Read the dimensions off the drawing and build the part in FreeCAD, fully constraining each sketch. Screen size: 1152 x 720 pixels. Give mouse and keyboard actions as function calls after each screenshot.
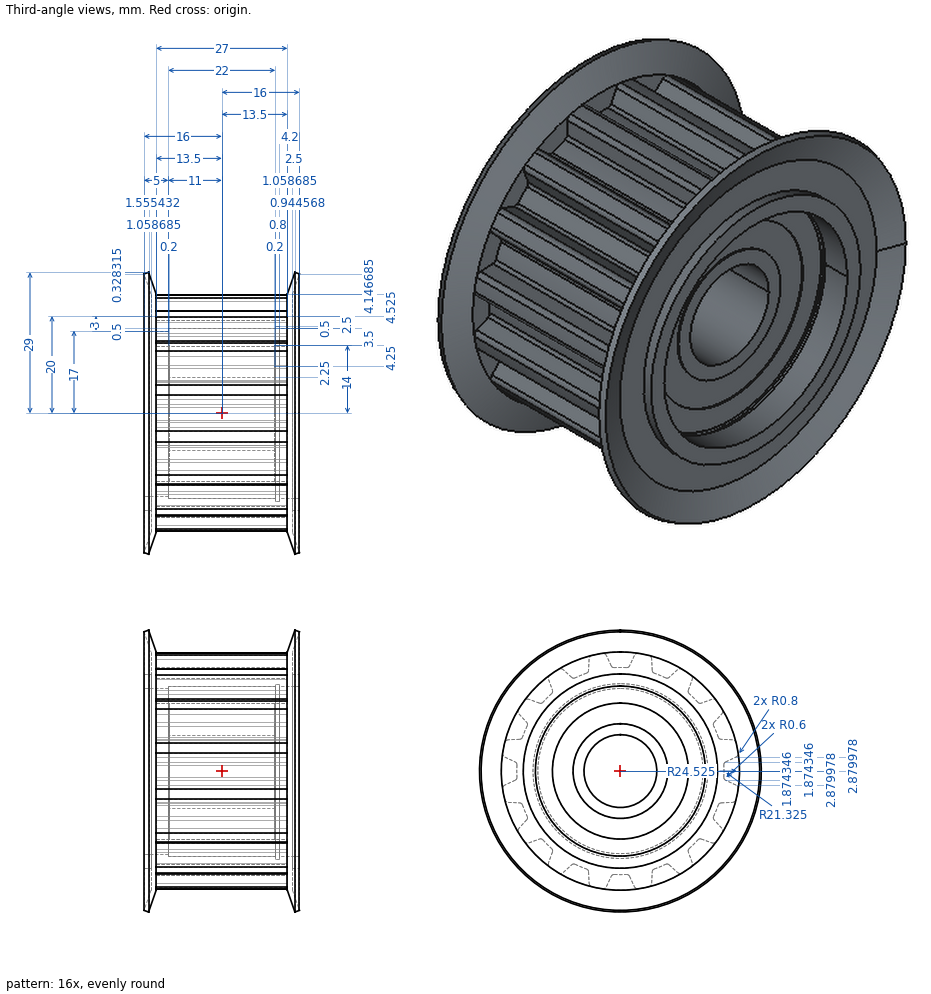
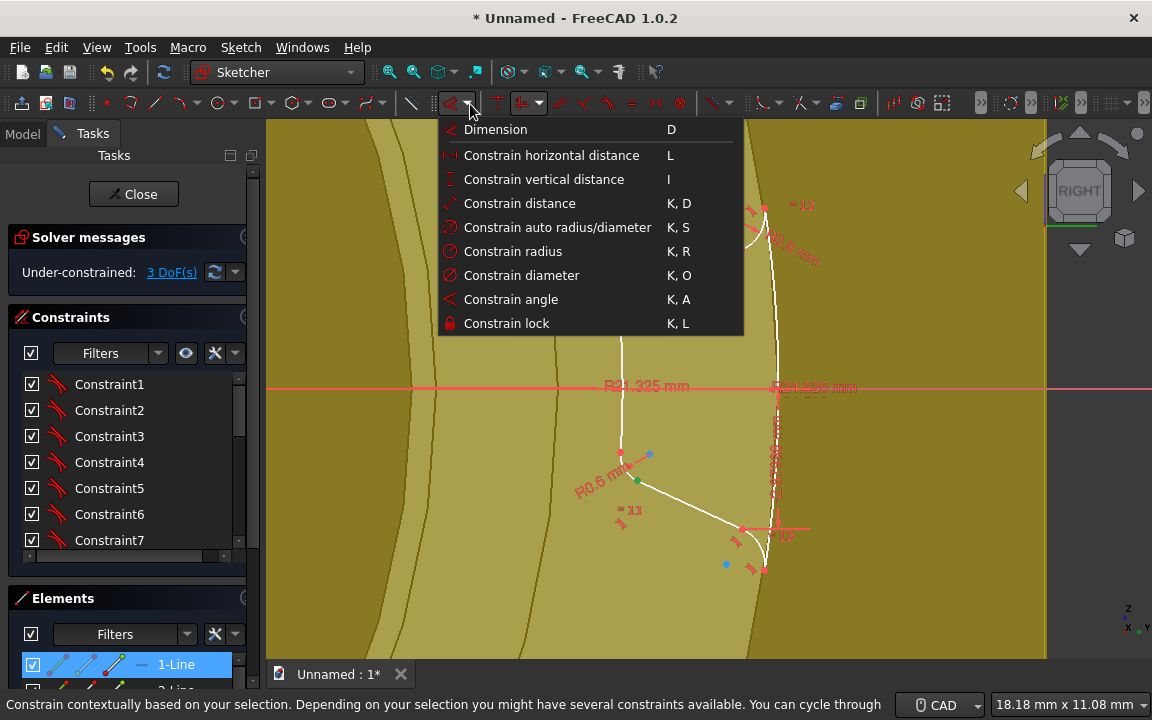
click(591, 179)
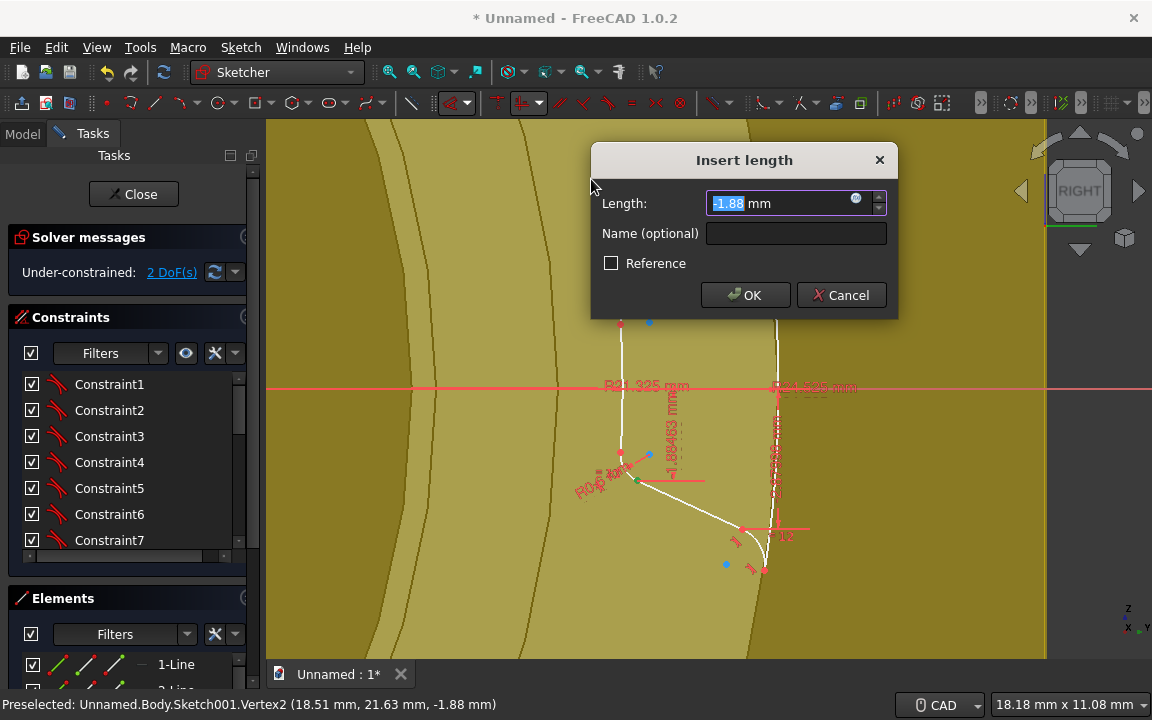
text(-1.874346)
key(Return)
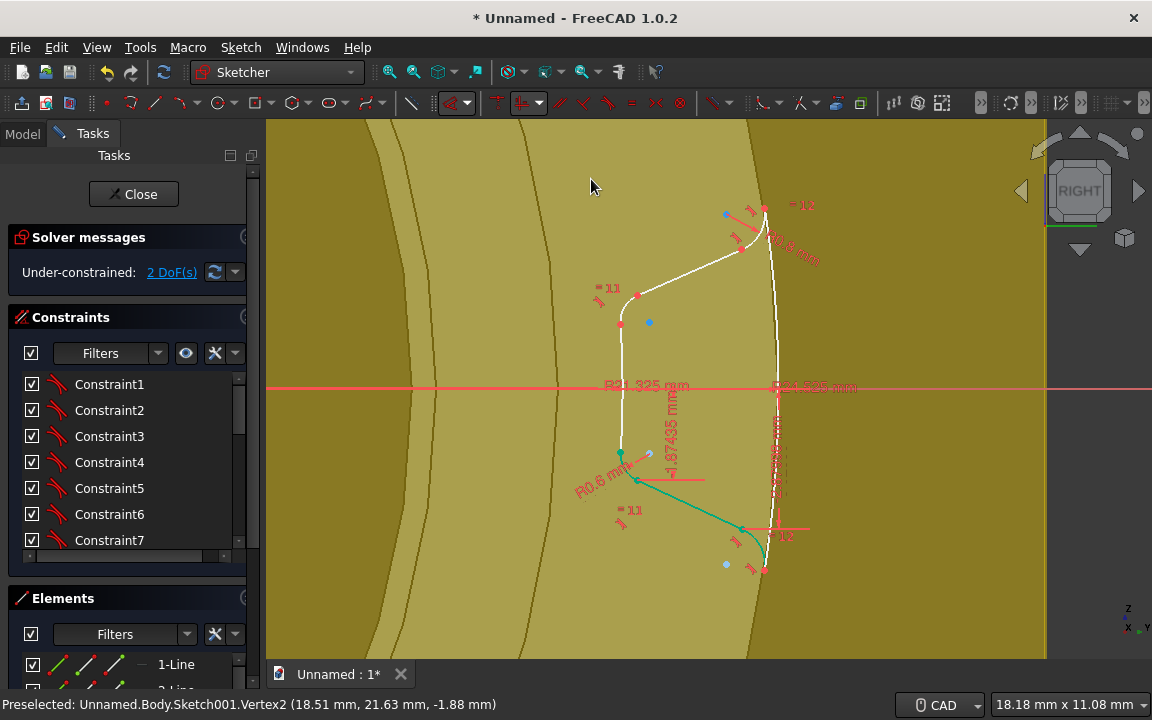
click(638, 295)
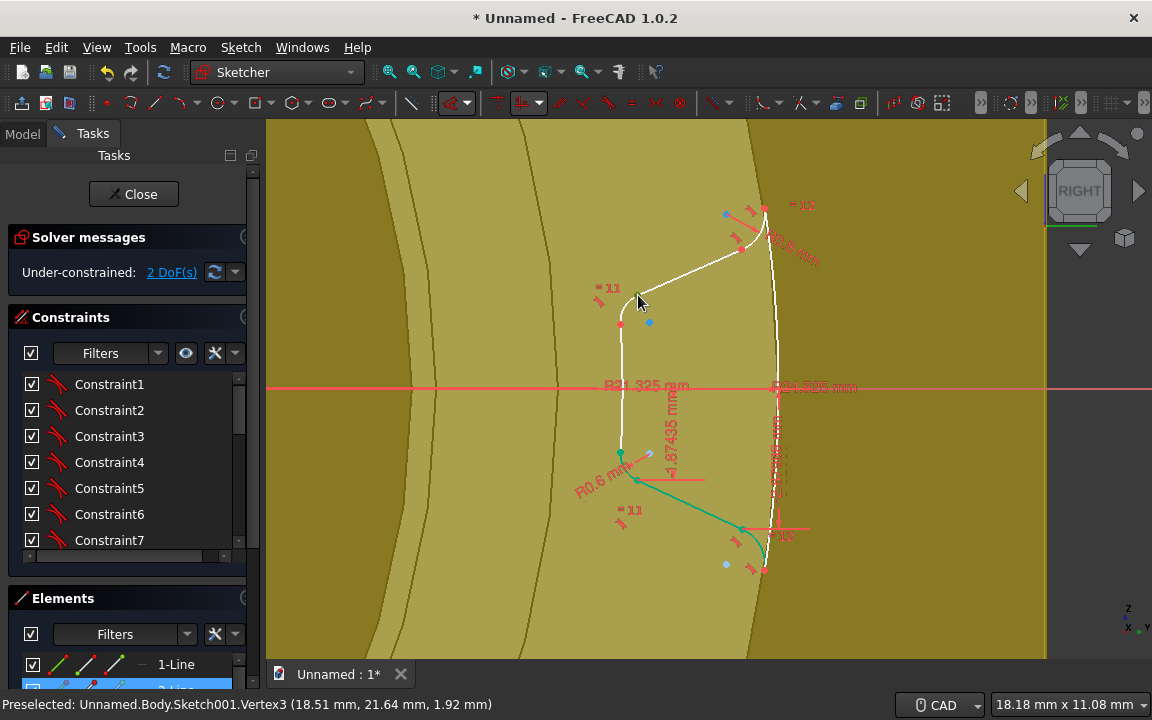
key(i)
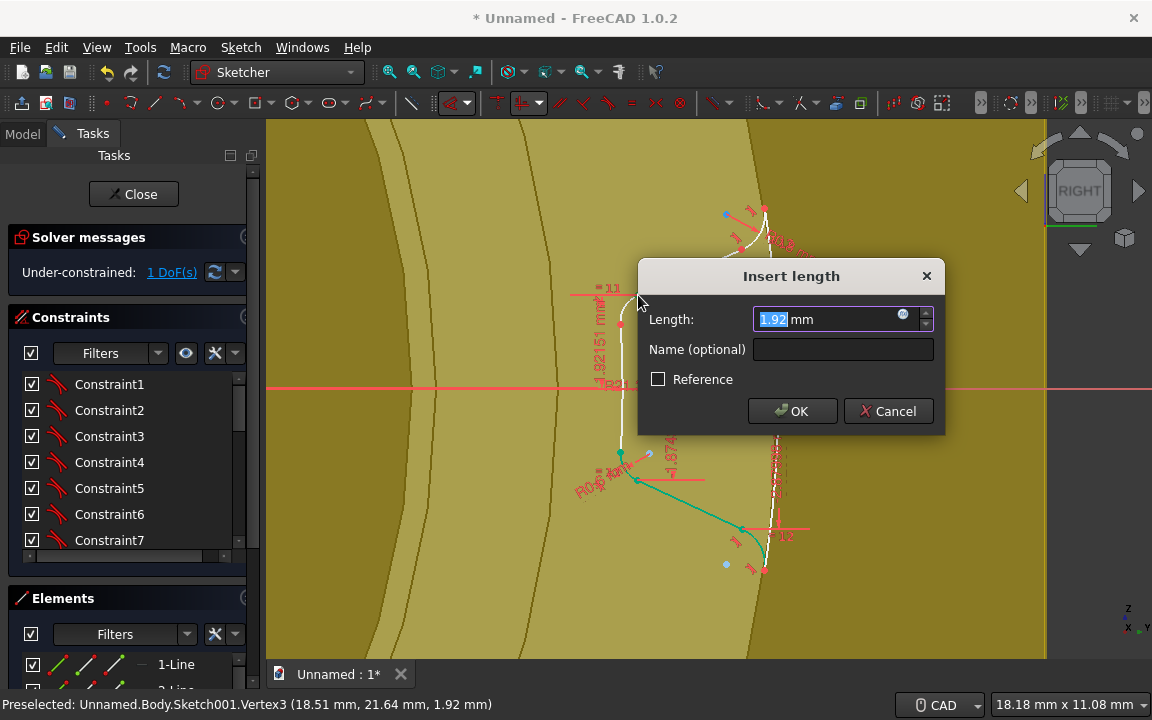
text(1.874346)
key(Return)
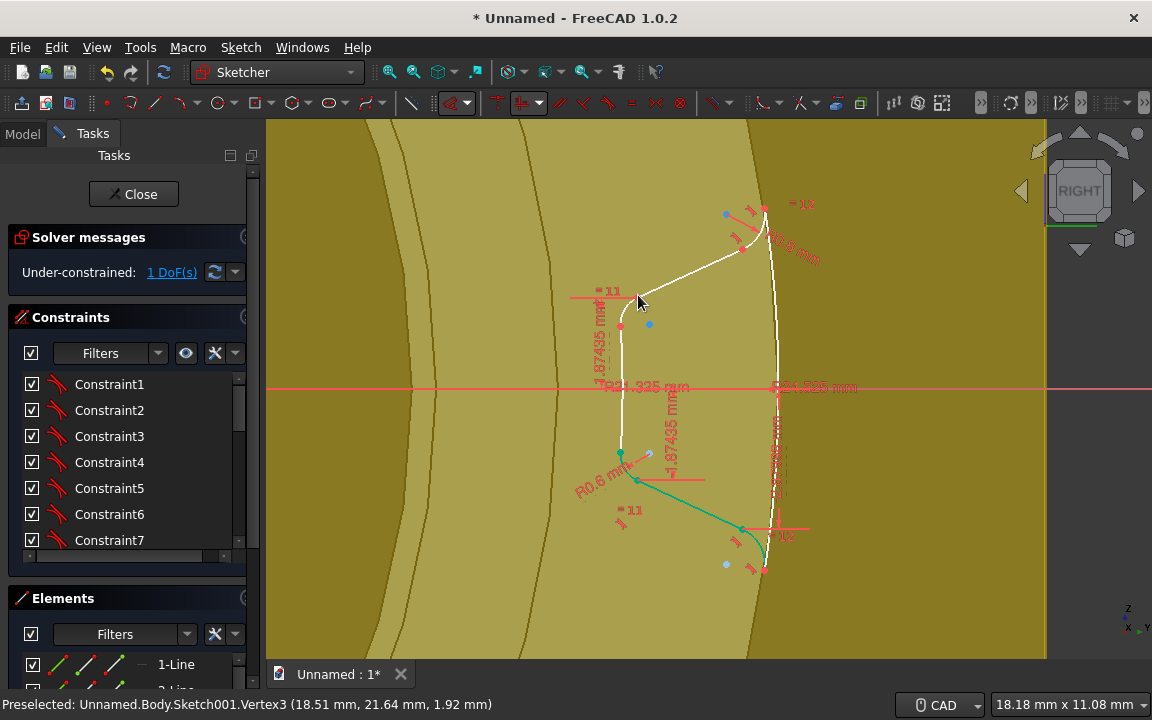
click(742, 250)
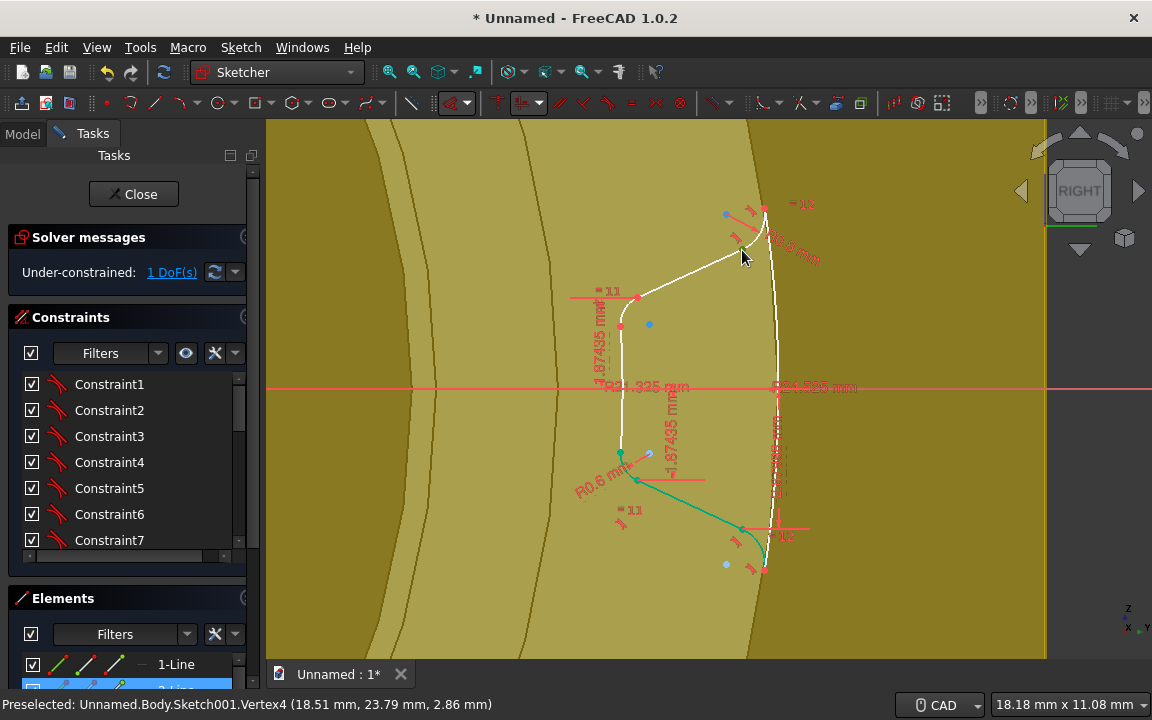
click(470, 104)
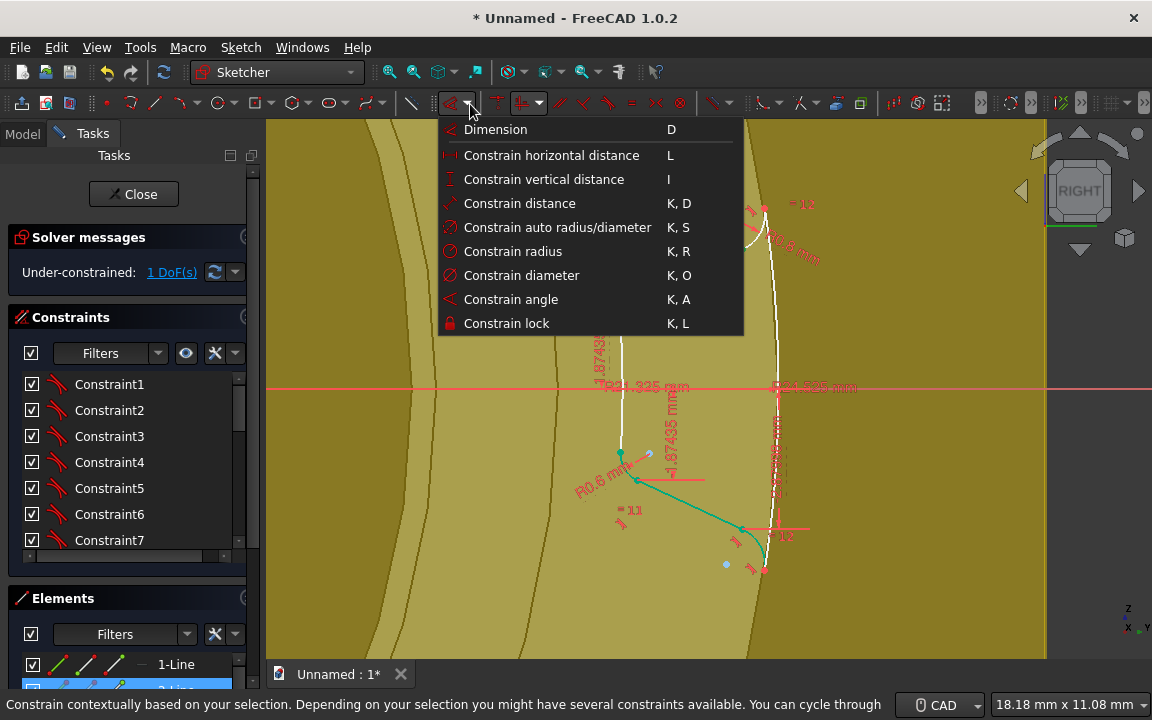
click(591, 179)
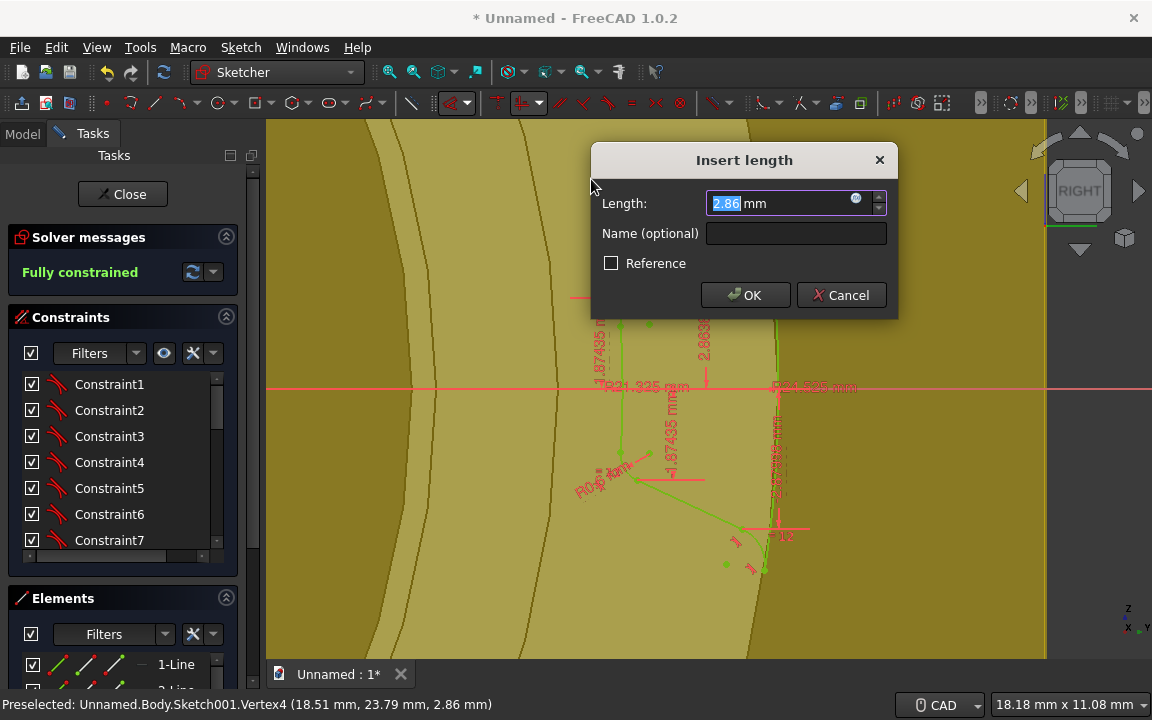
text(2.879978)
key(Return)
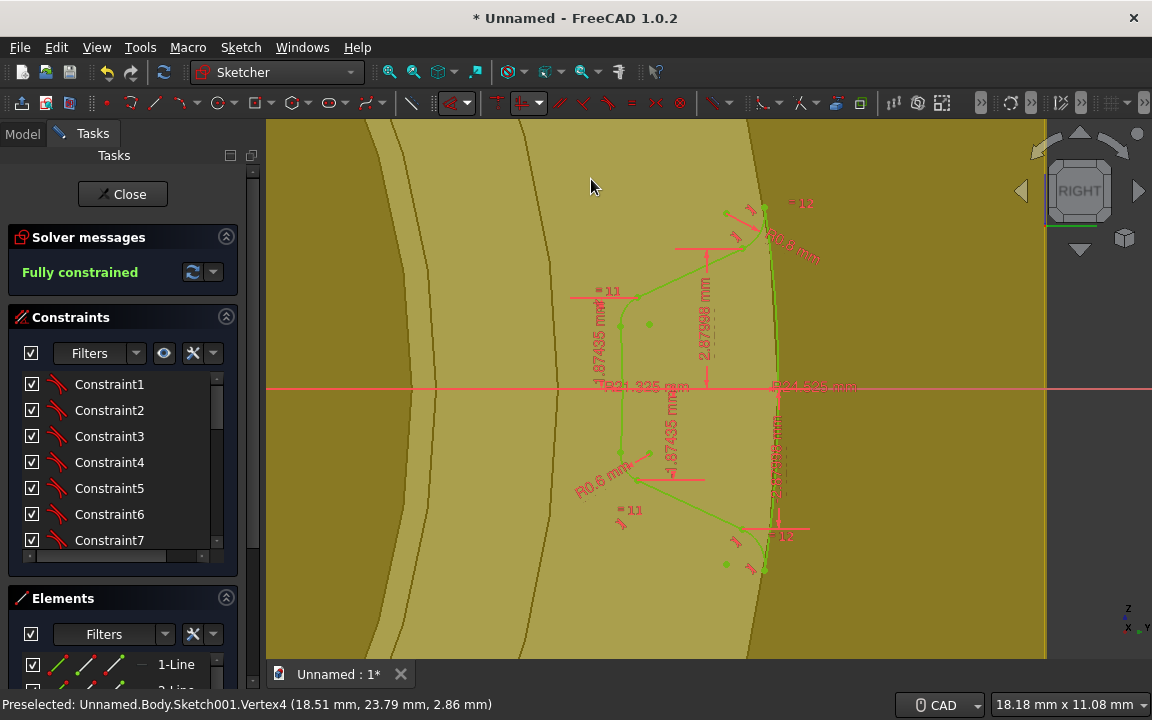
click(123, 194)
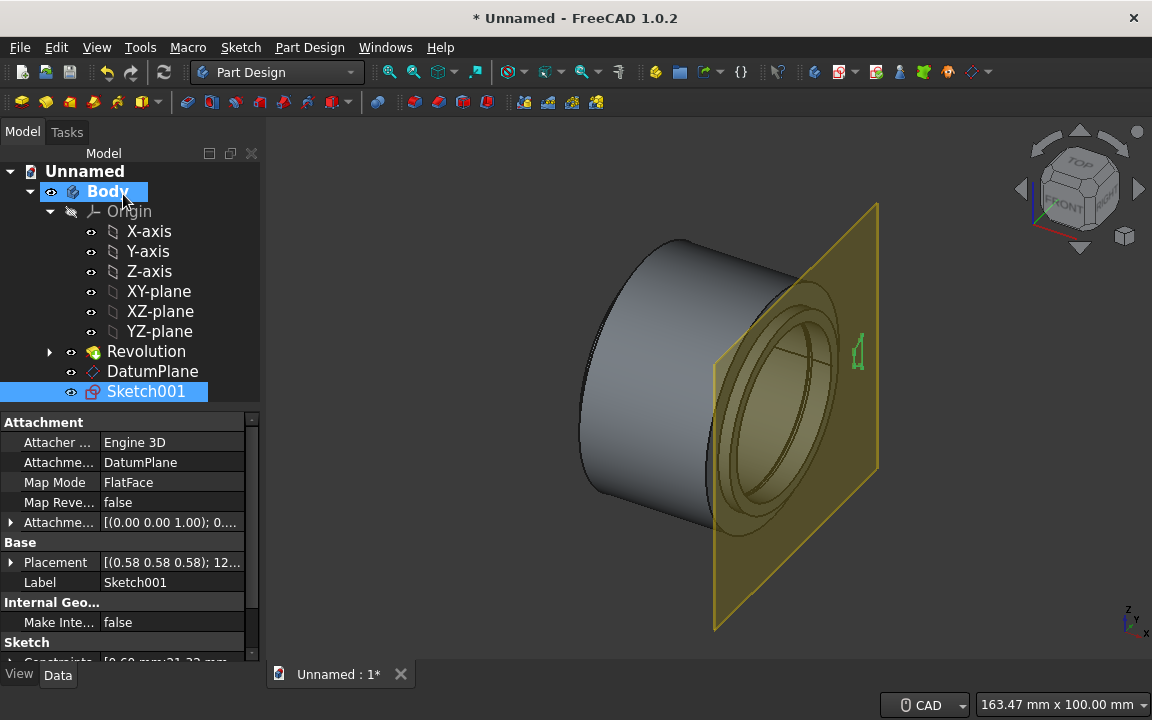
click(188, 102)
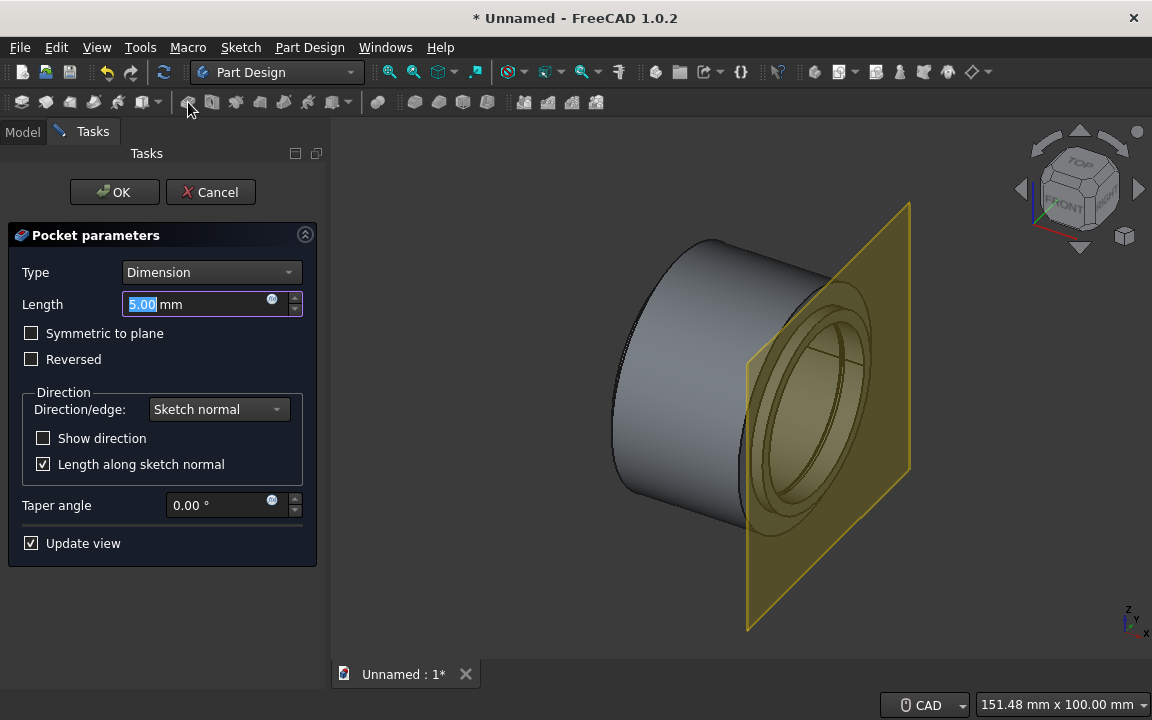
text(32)
key(Tab)